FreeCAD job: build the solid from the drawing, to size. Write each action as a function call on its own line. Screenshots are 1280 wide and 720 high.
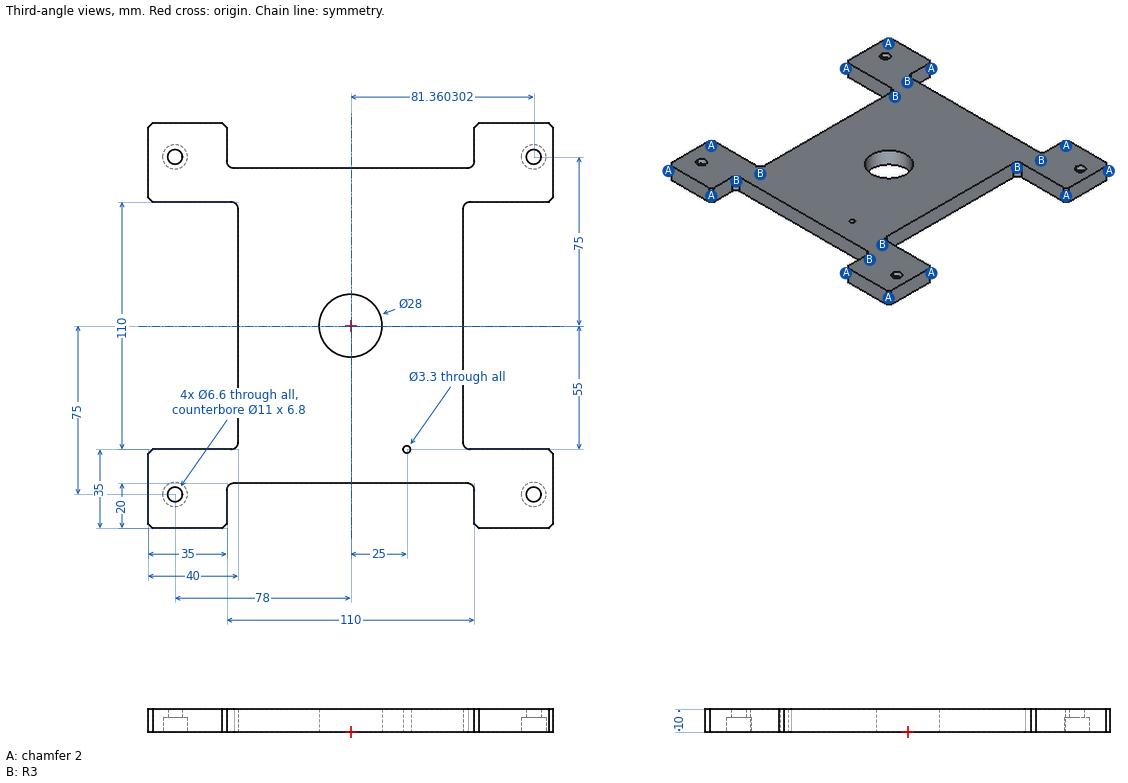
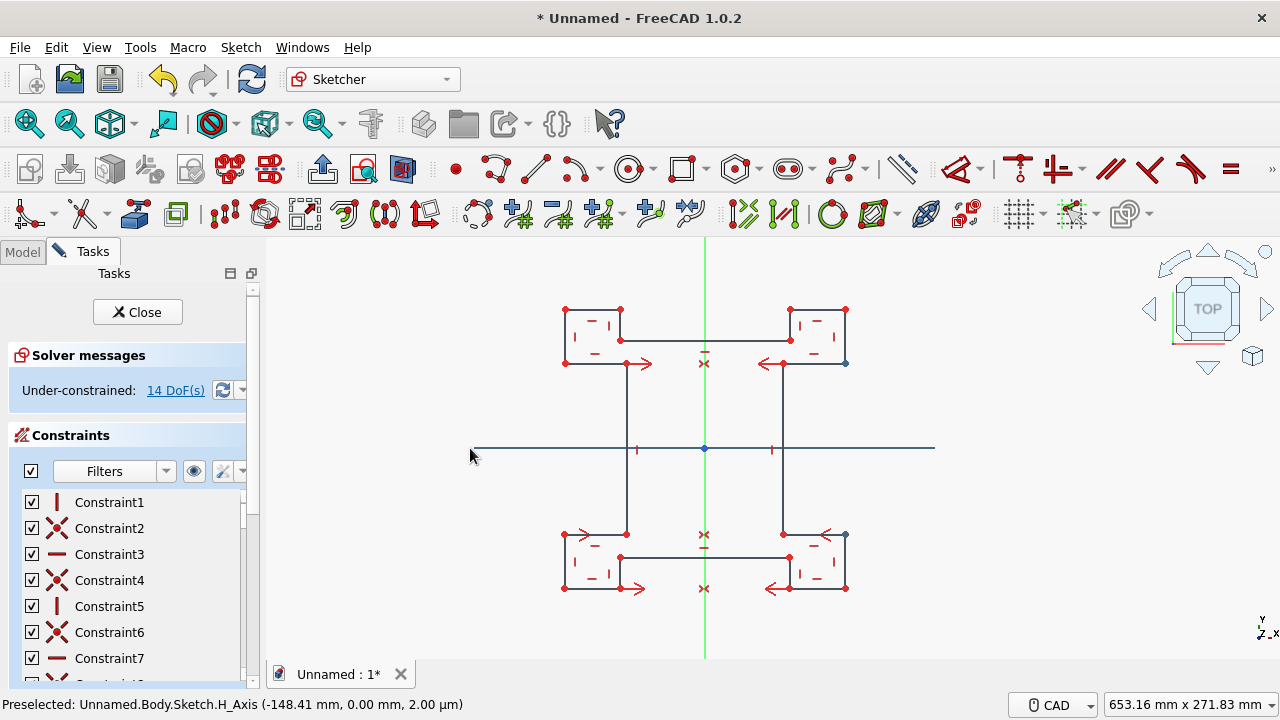
key(s)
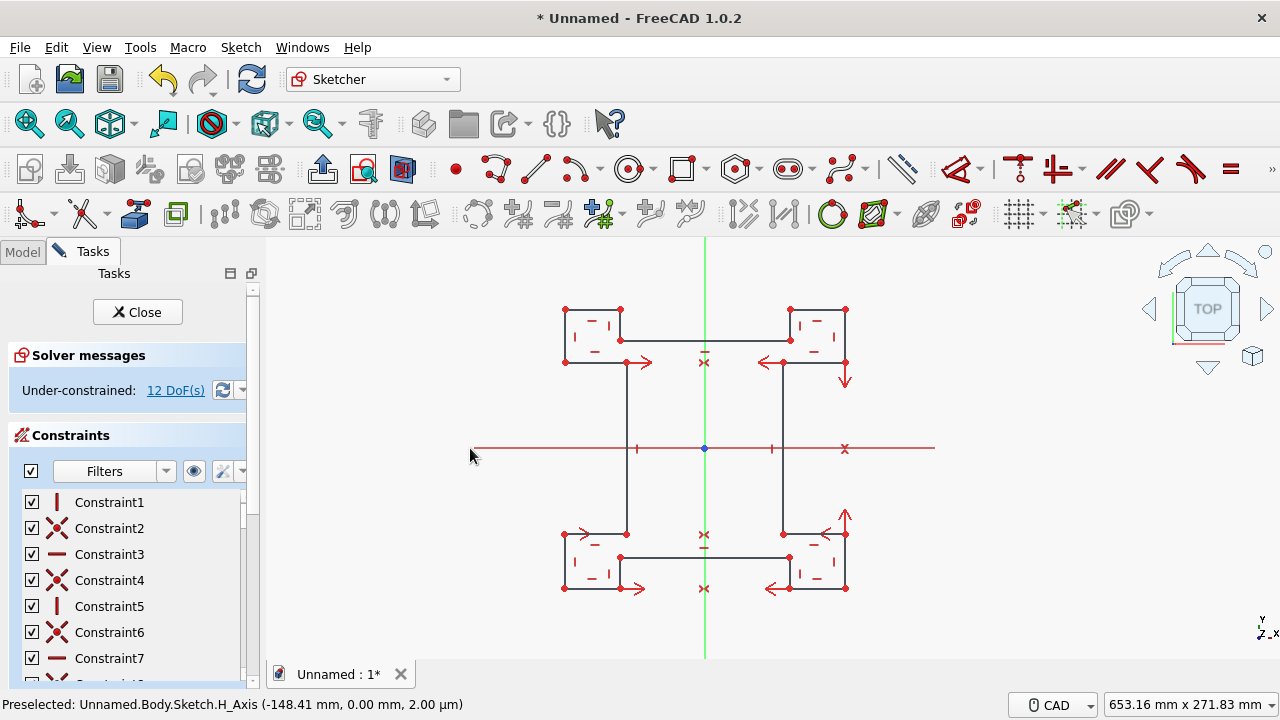
click(790, 589)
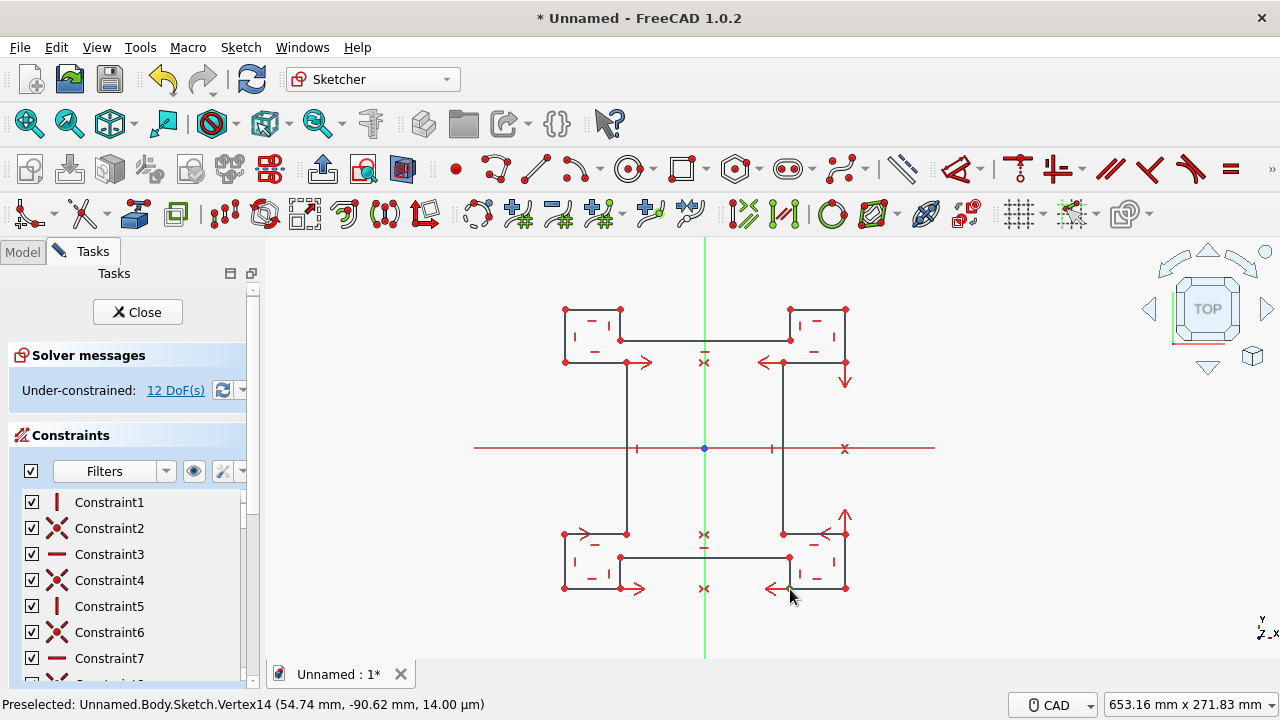
click(790, 310)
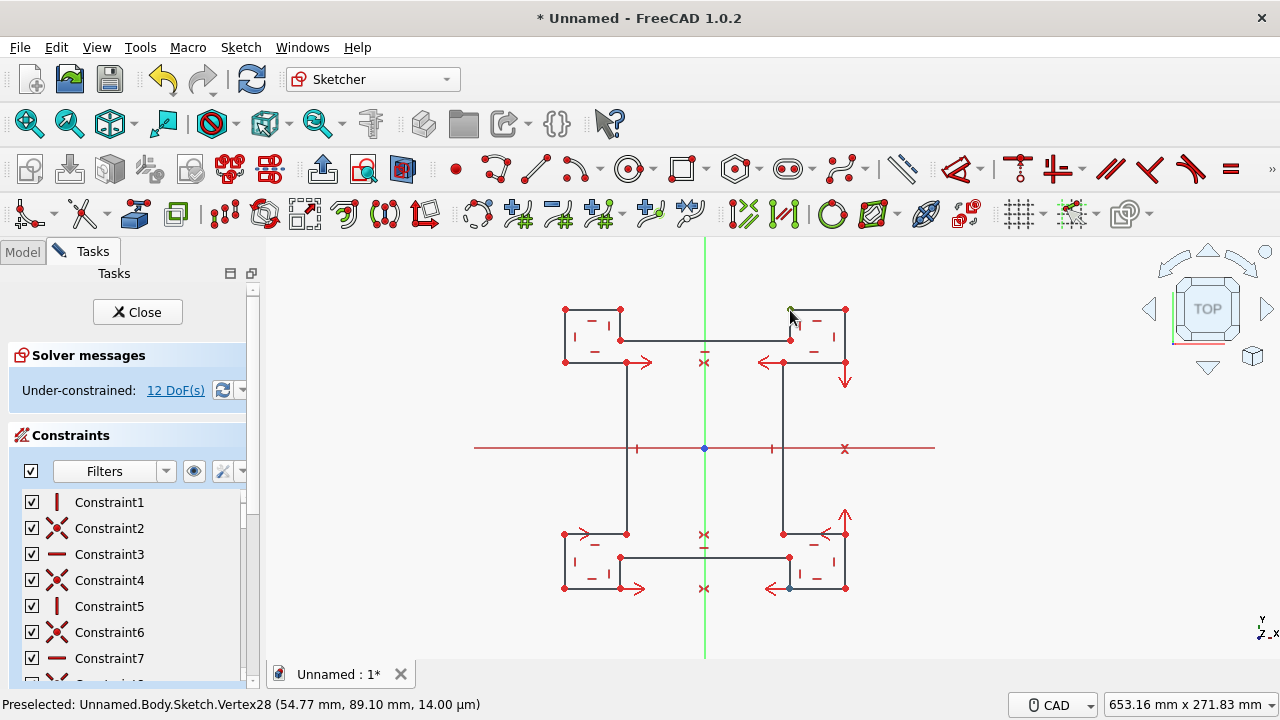
click(470, 448)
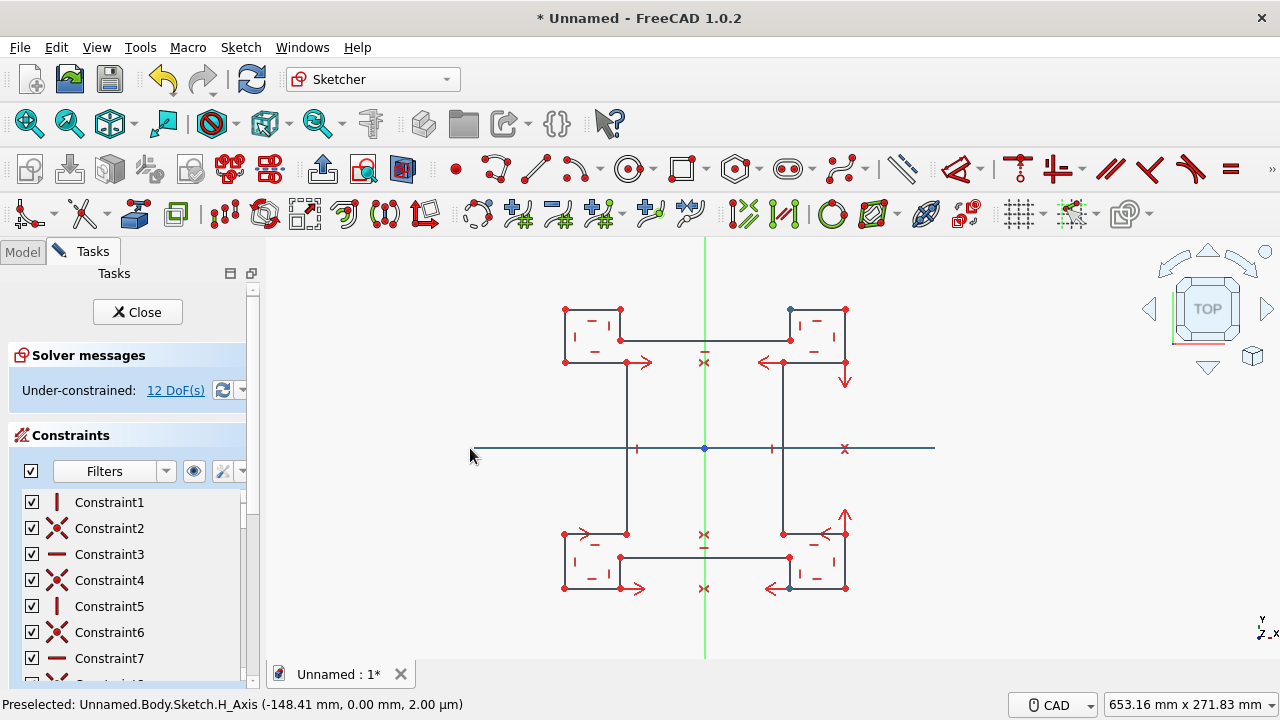
key(s)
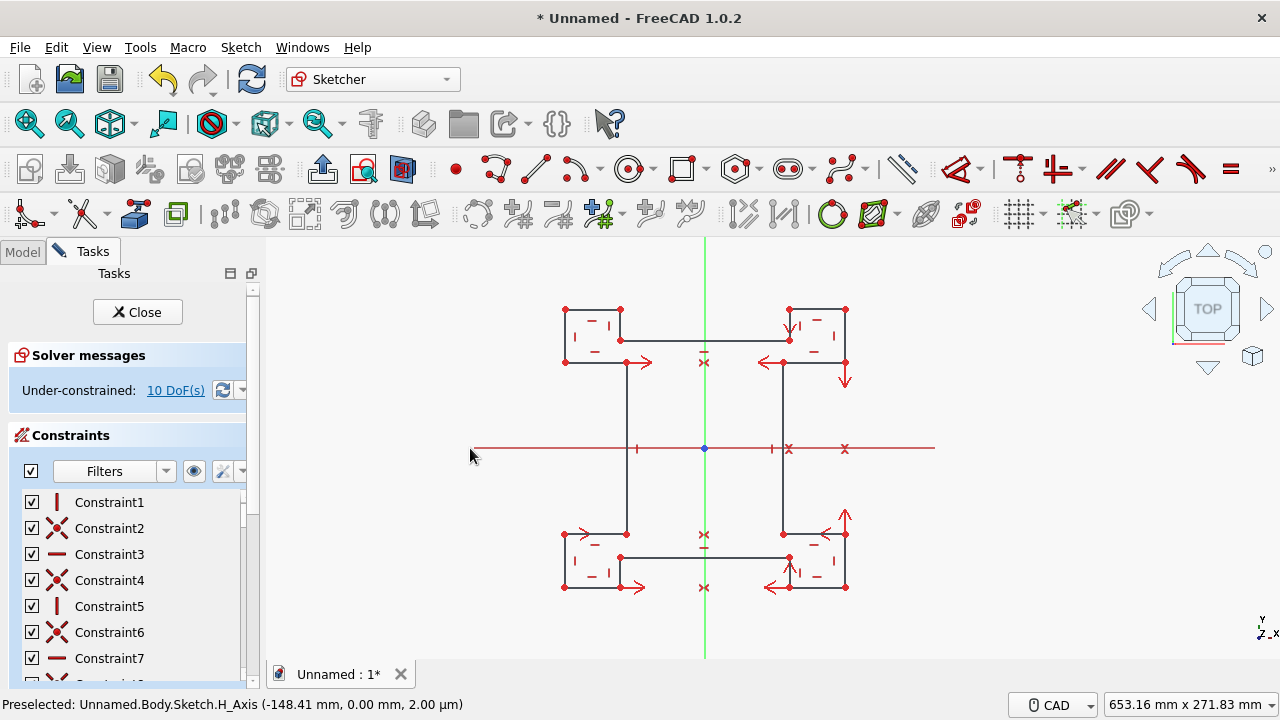
click(620, 558)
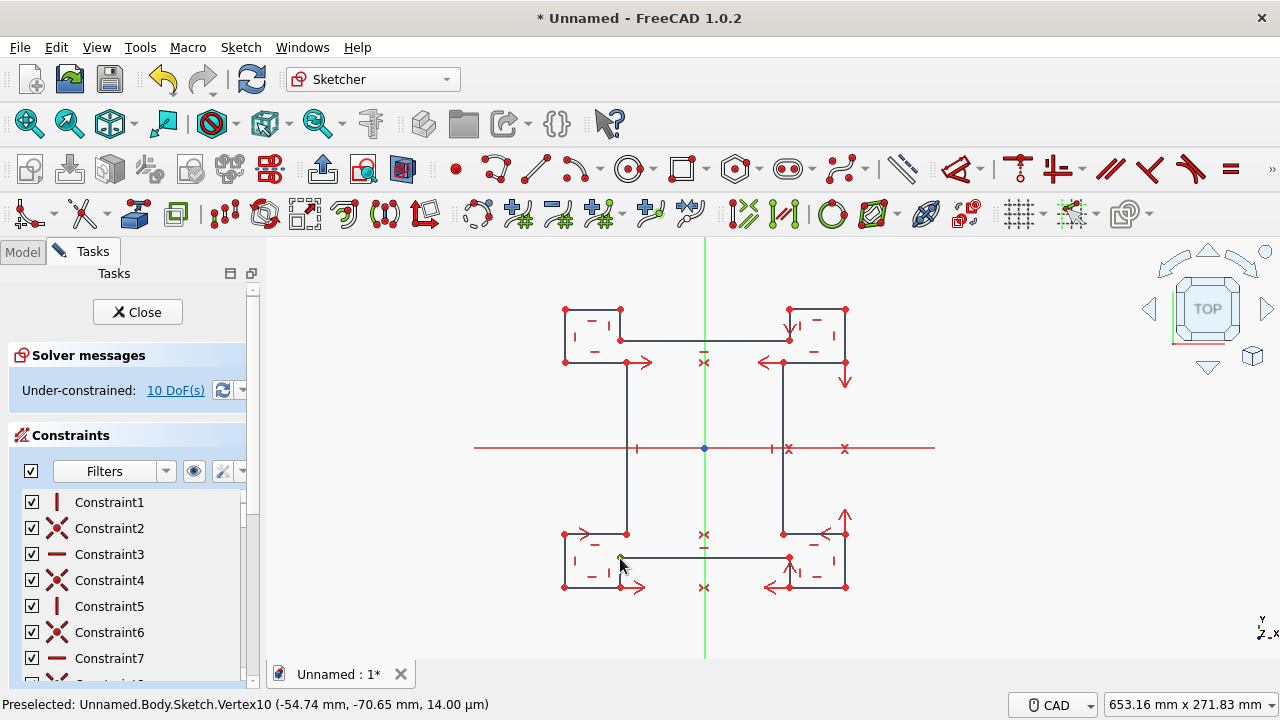
click(620, 341)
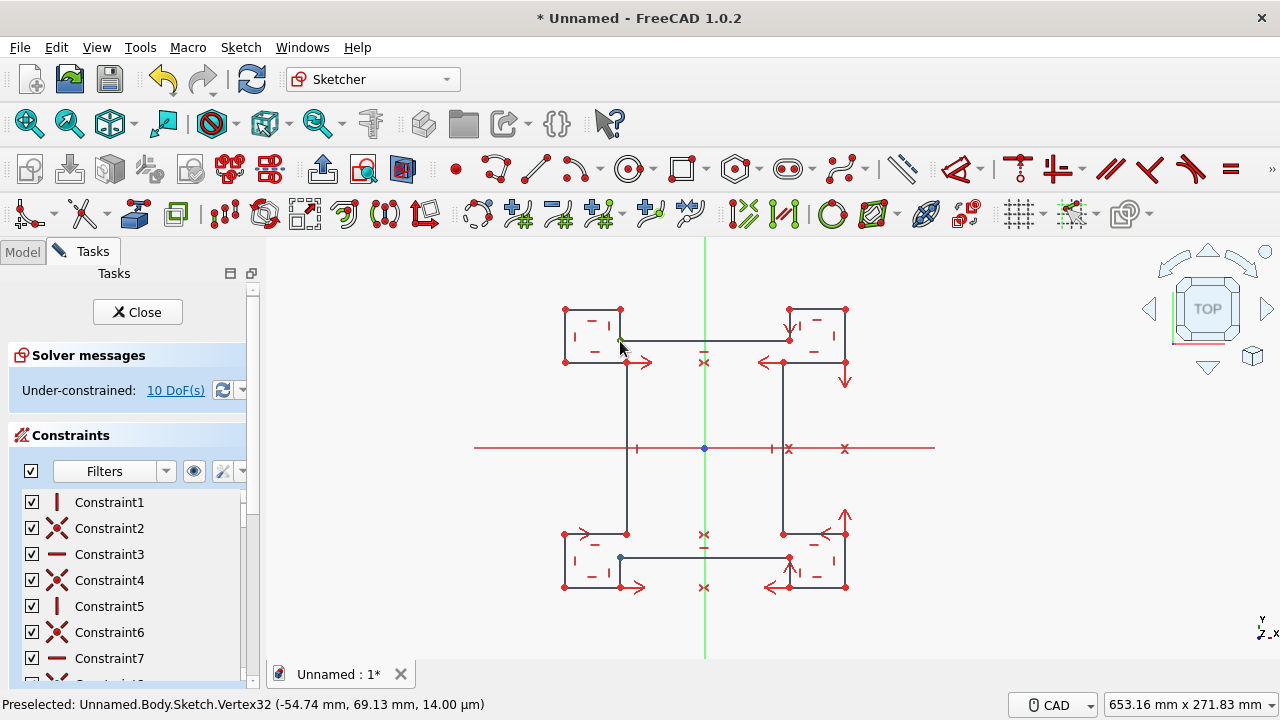
click(470, 448)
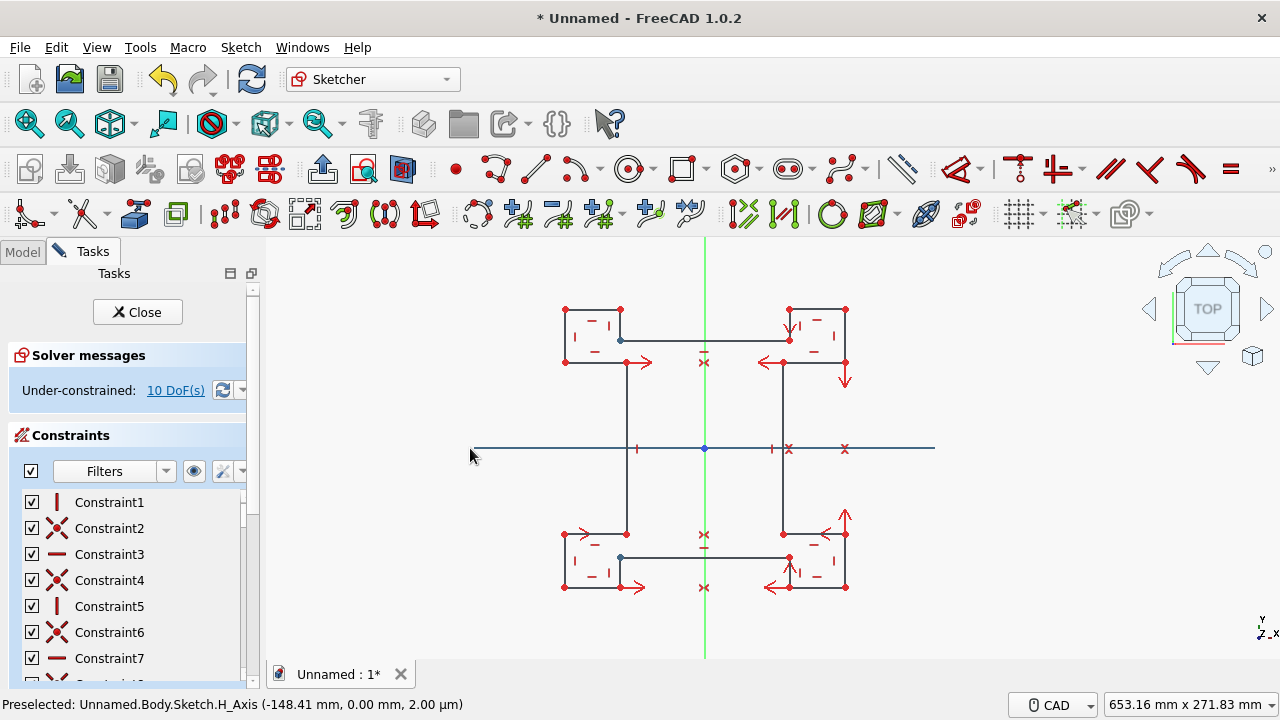
key(s)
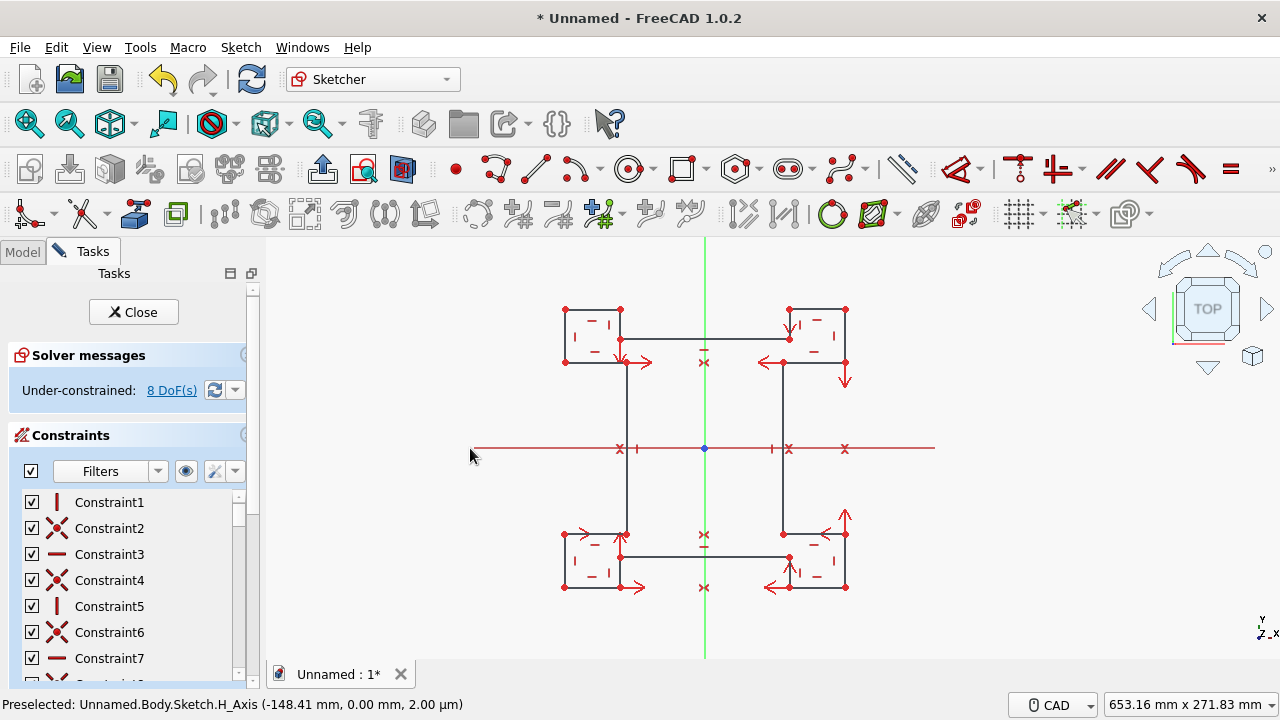
click(565, 588)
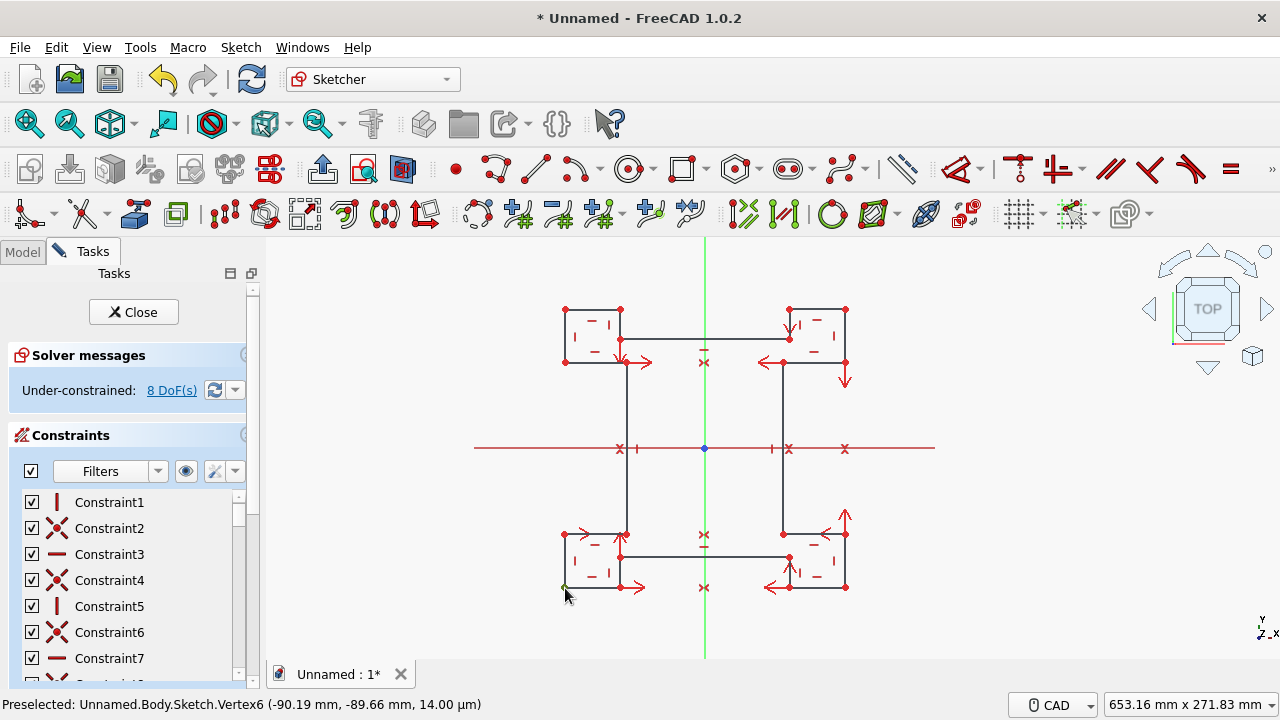
click(565, 310)